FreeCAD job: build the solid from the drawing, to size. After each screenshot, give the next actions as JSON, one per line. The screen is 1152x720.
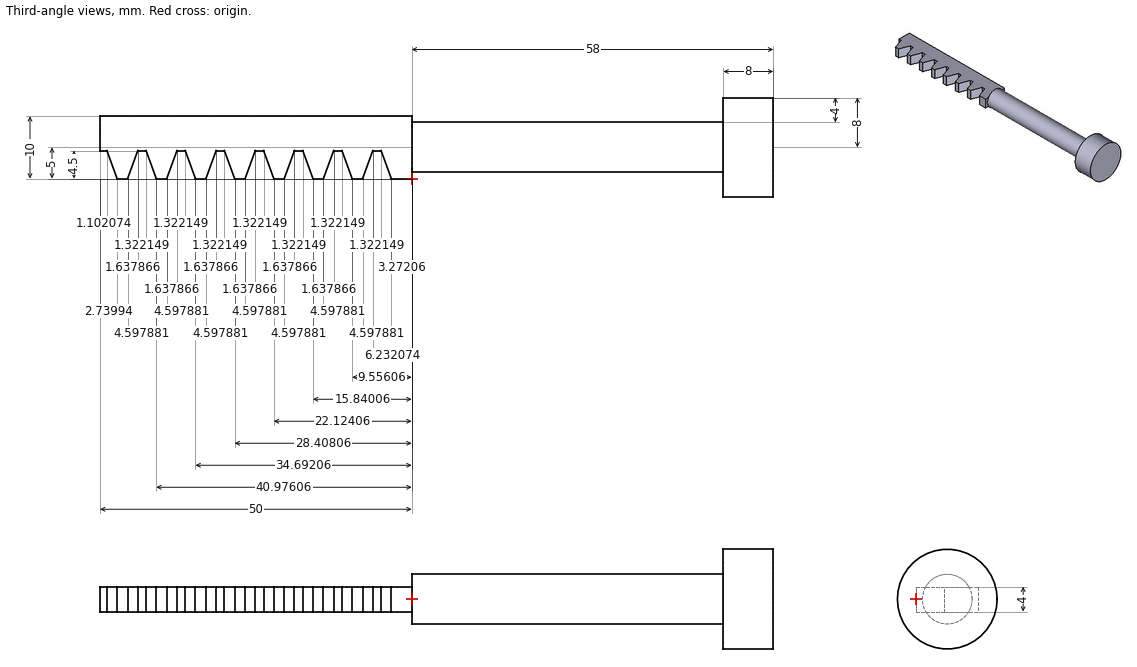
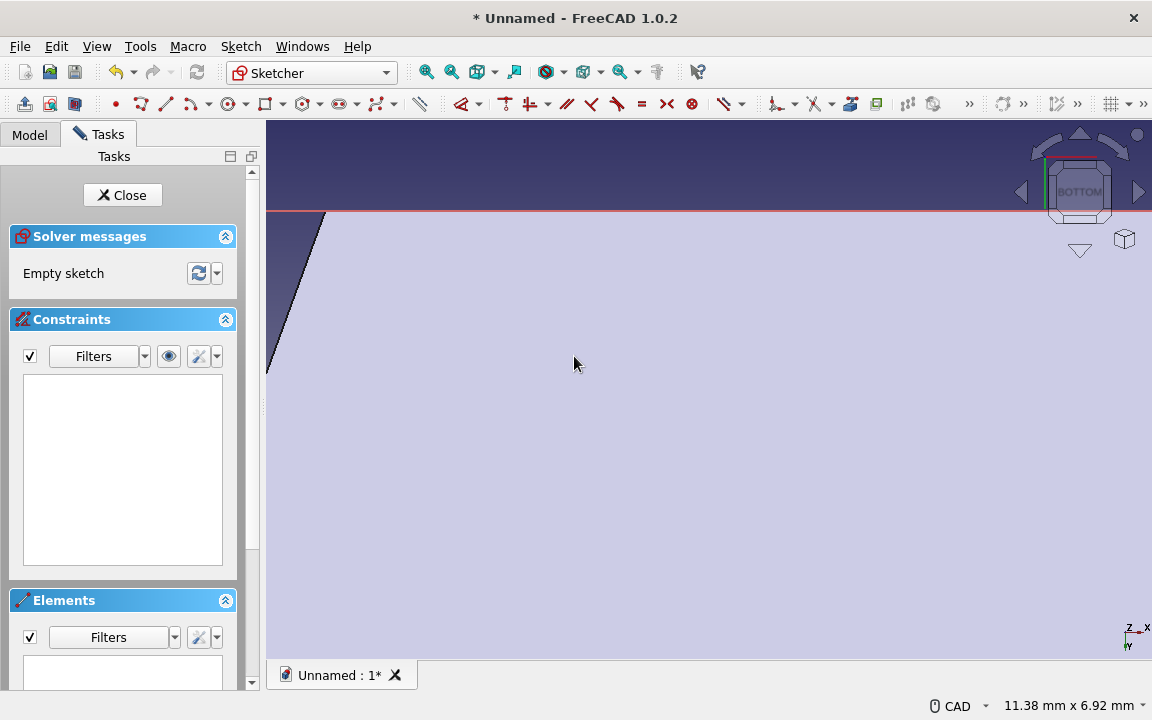
{"action": "left_click", "coordinate": [141, 104]}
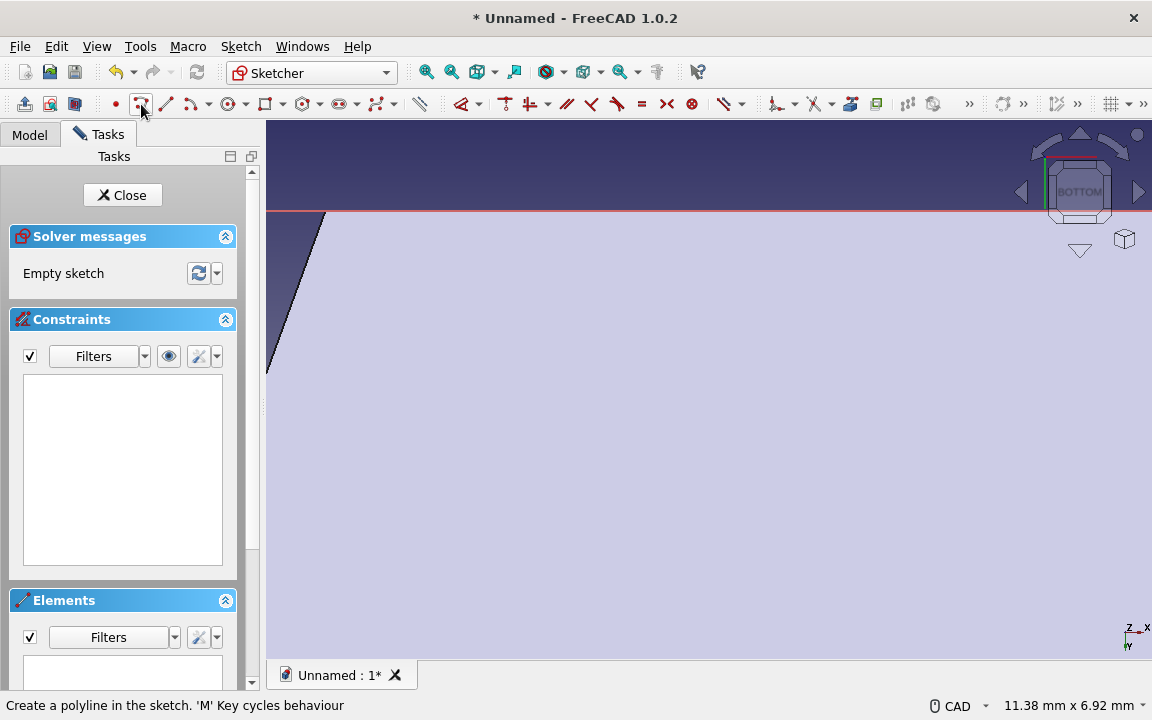
{"action": "left_click", "coordinate": [815, 211]}
{"action": "left_click", "coordinate": [457, 220]}
{"action": "left_click", "coordinate": [584, 562]}
{"action": "left_click", "coordinate": [687, 562]}
{"action": "left_click", "coordinate": [815, 211]}
{"action": "key", "text": "Escape"}
{"action": "key", "text": "Escape"}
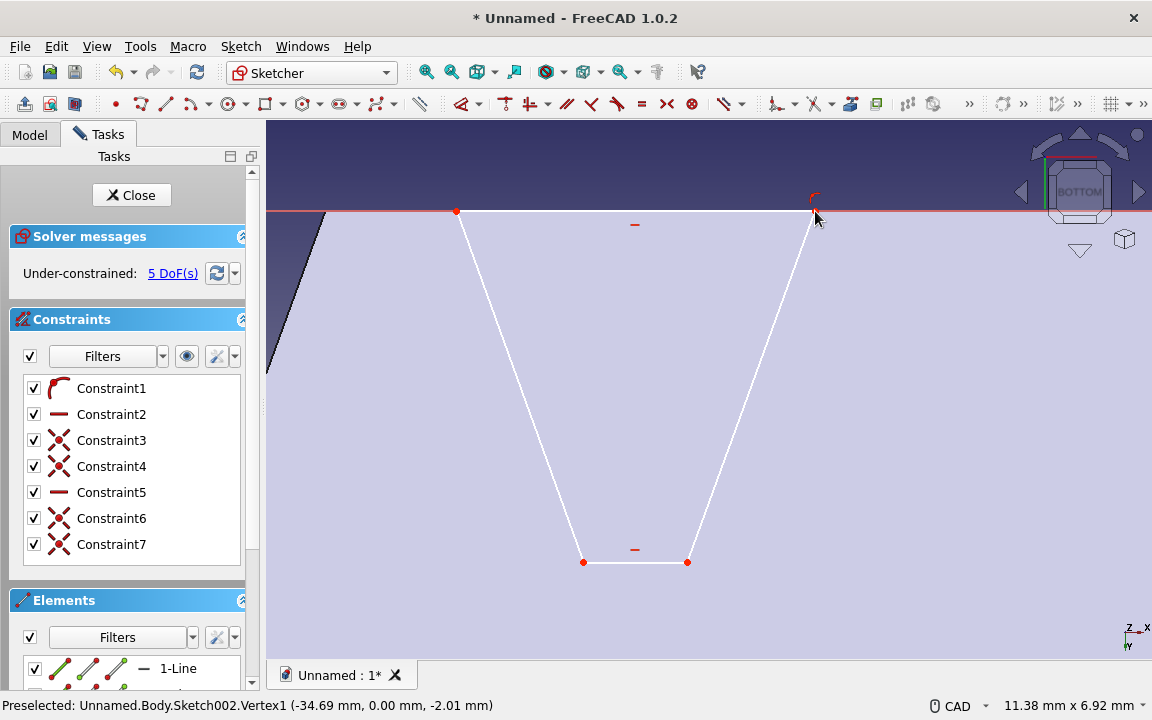
{"action": "left_click", "coordinate": [460, 104]}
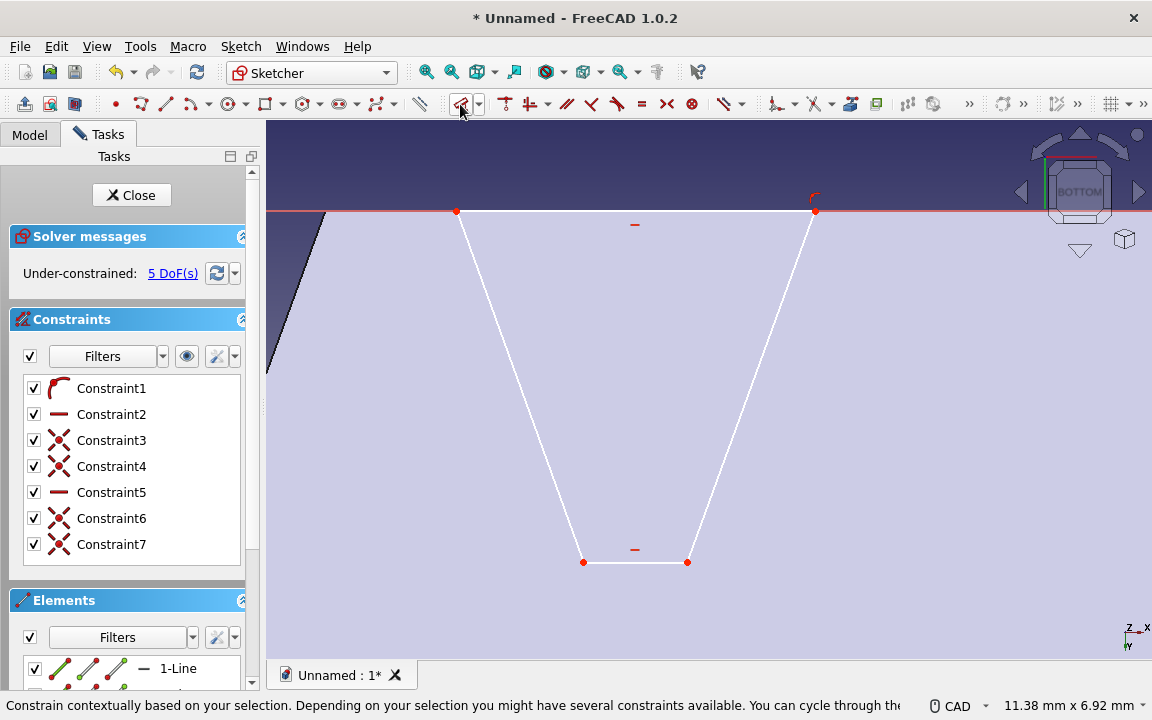
{"action": "left_click", "coordinate": [584, 563]}
{"action": "left_click", "coordinate": [550, 387]}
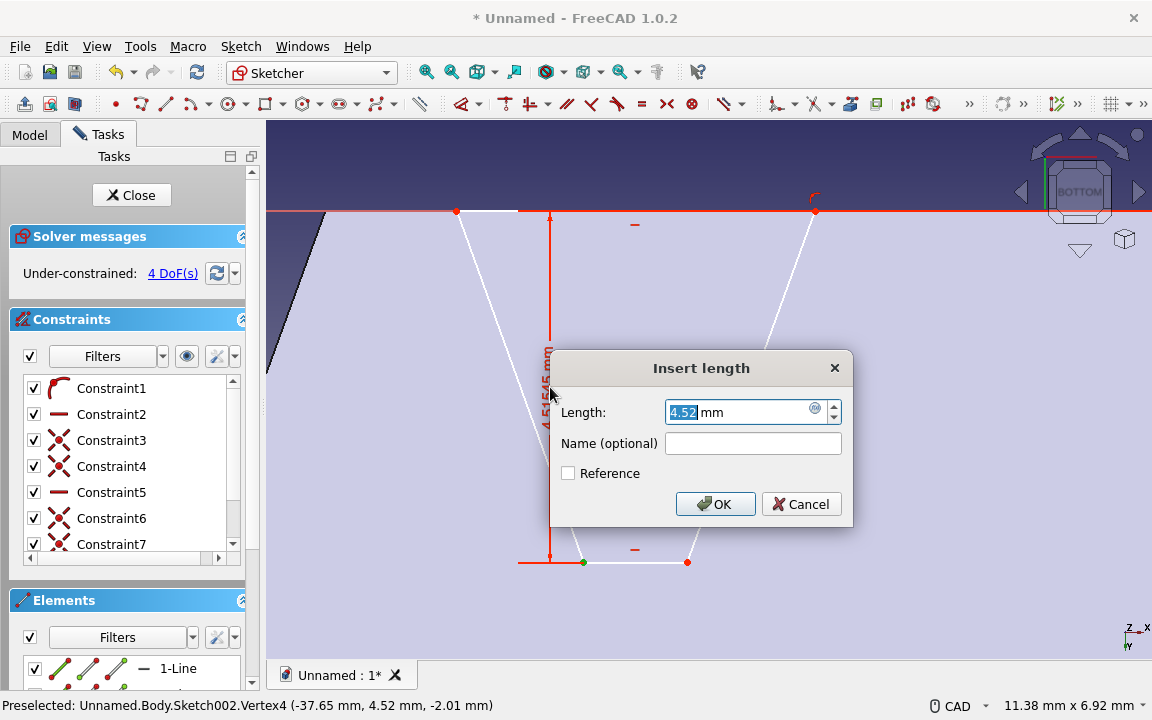
{"action": "type", "text": "4.5"}
{"action": "key", "text": "Return"}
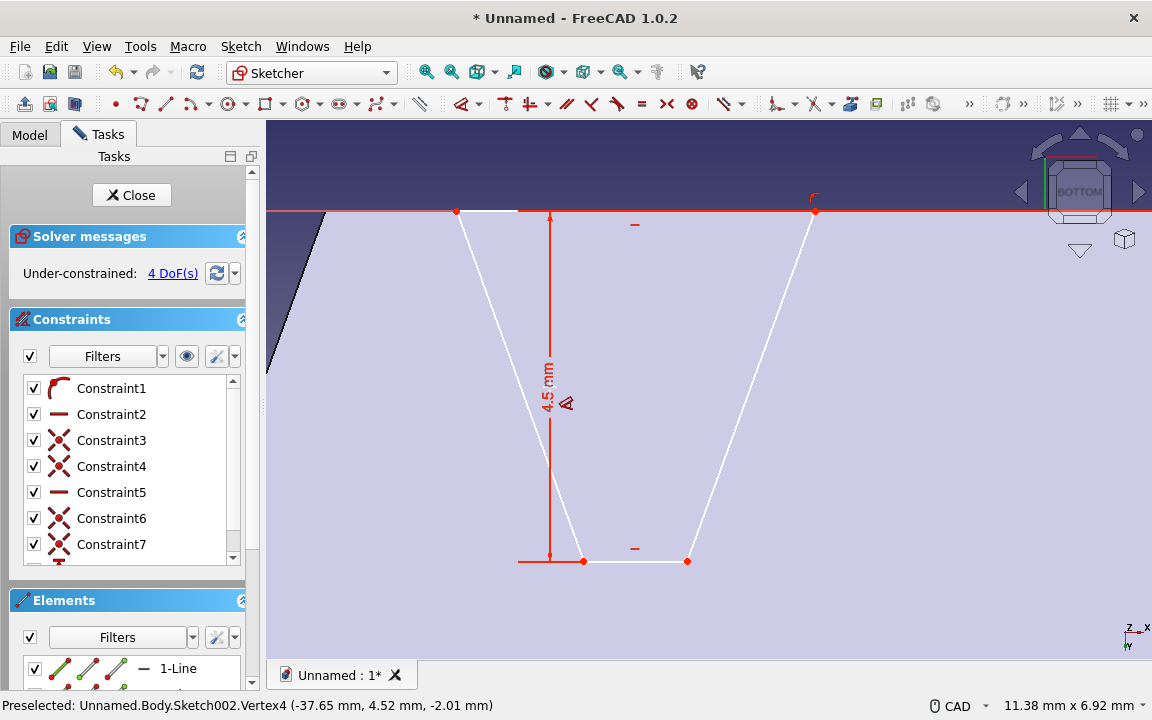
{"action": "left_click", "coordinate": [708, 211]}
{"action": "left_click", "coordinate": [636, 177]}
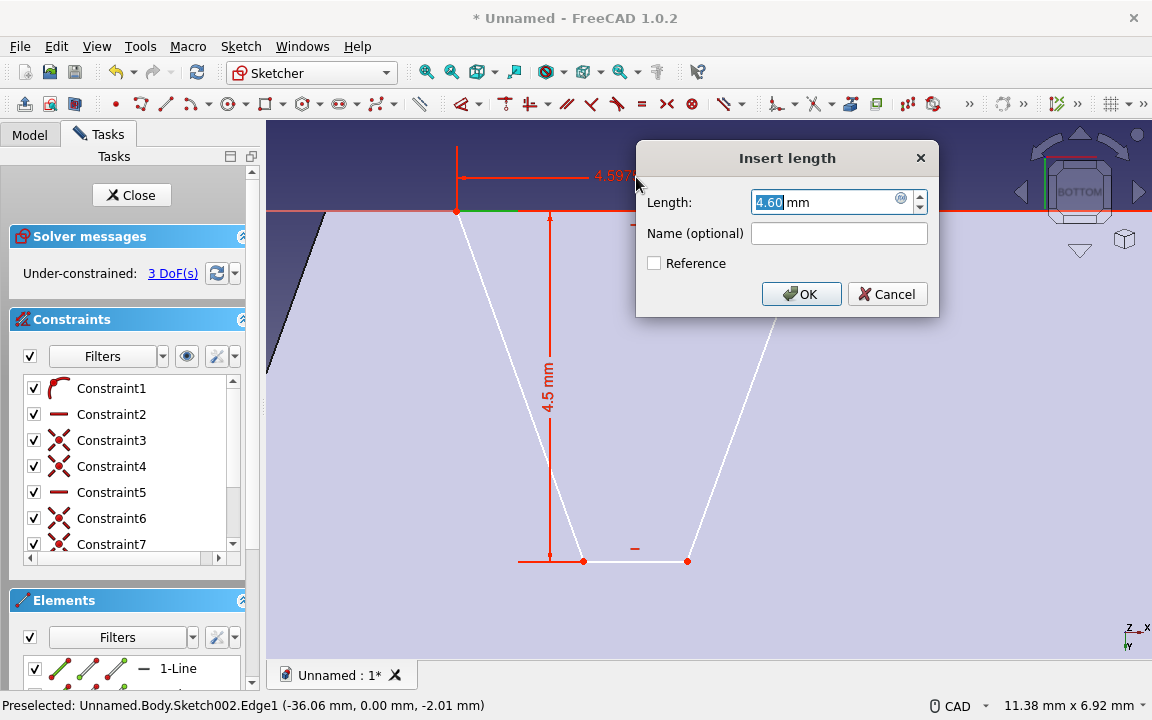
{"action": "type", "text": "4.597881"}
{"action": "key", "text": "Return"}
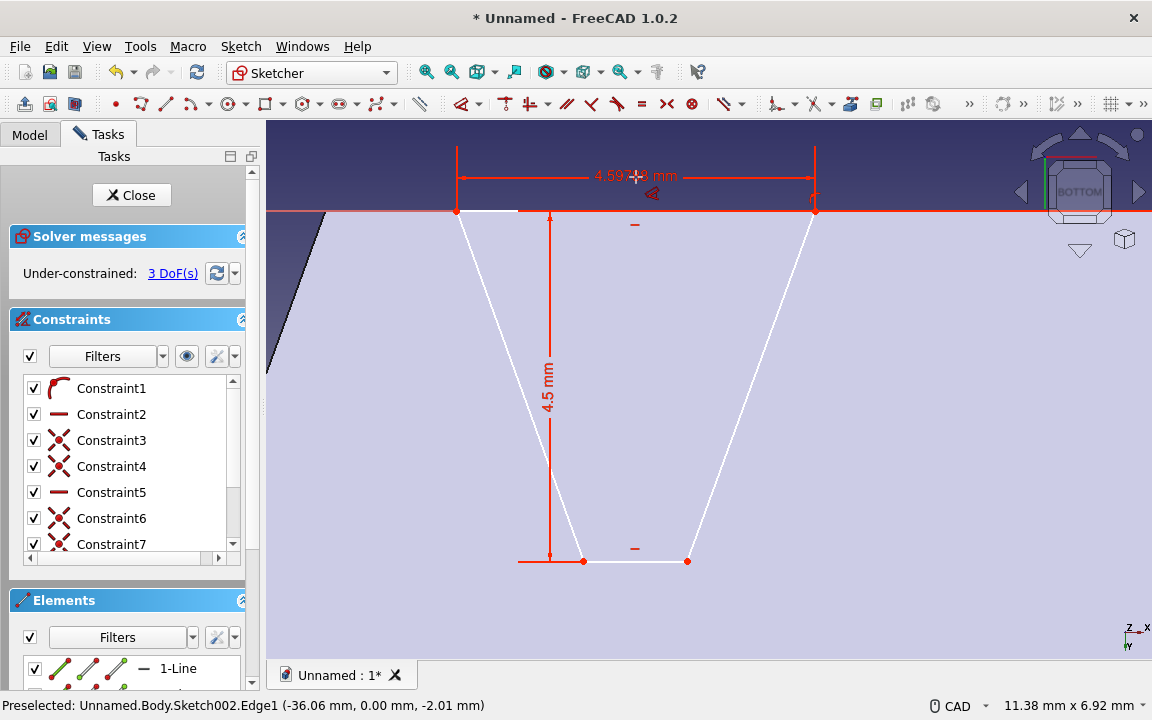
{"action": "left_click", "coordinate": [615, 562]}
{"action": "left_click", "coordinate": [636, 596]}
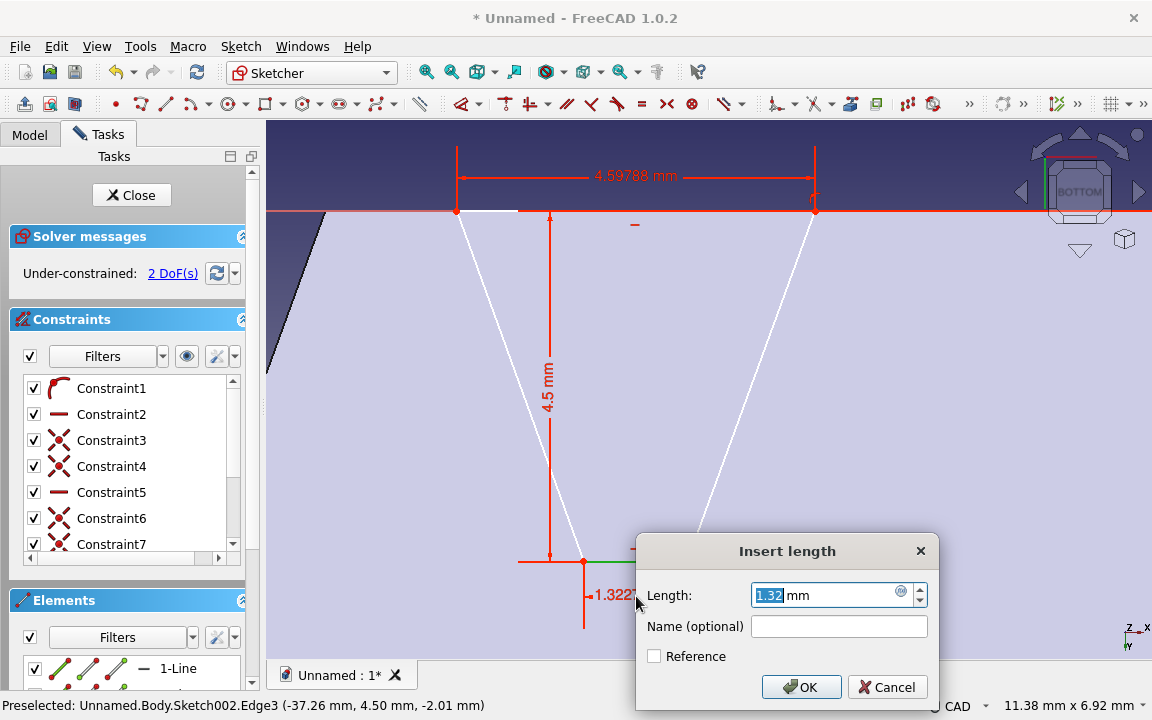
{"action": "type", "text": "1.322149"}
{"action": "key", "text": "Return"}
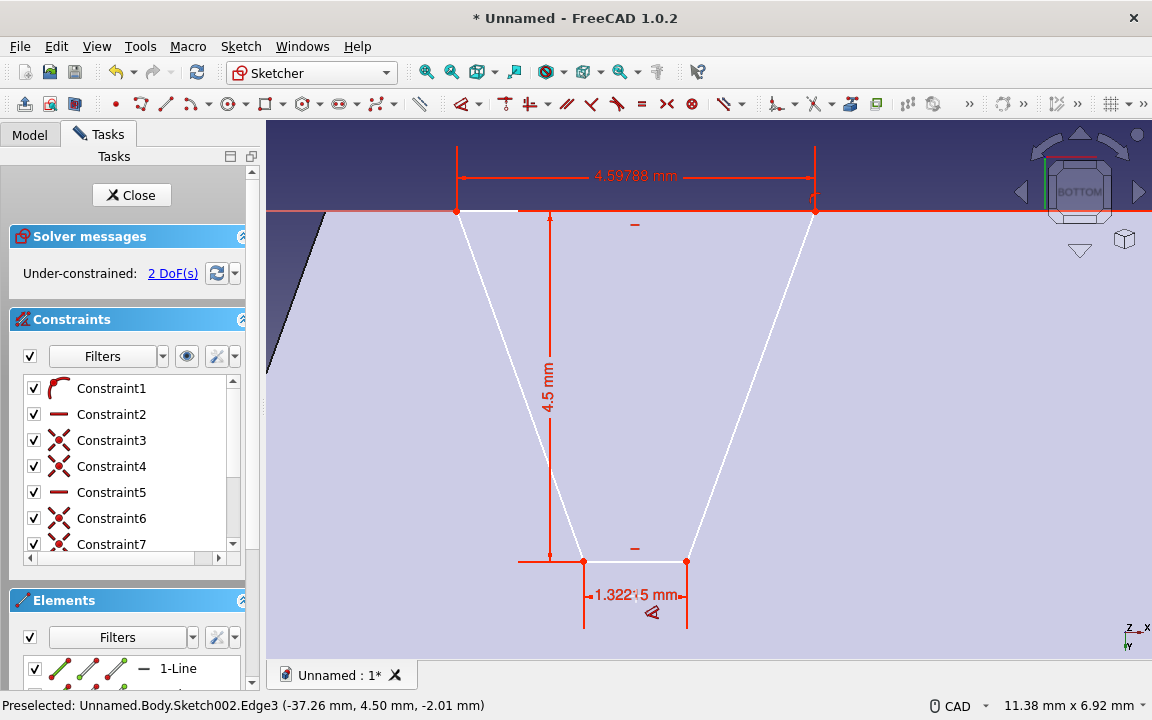
{"action": "left_click", "coordinate": [815, 211]}
{"action": "left_click", "coordinate": [901, 177]}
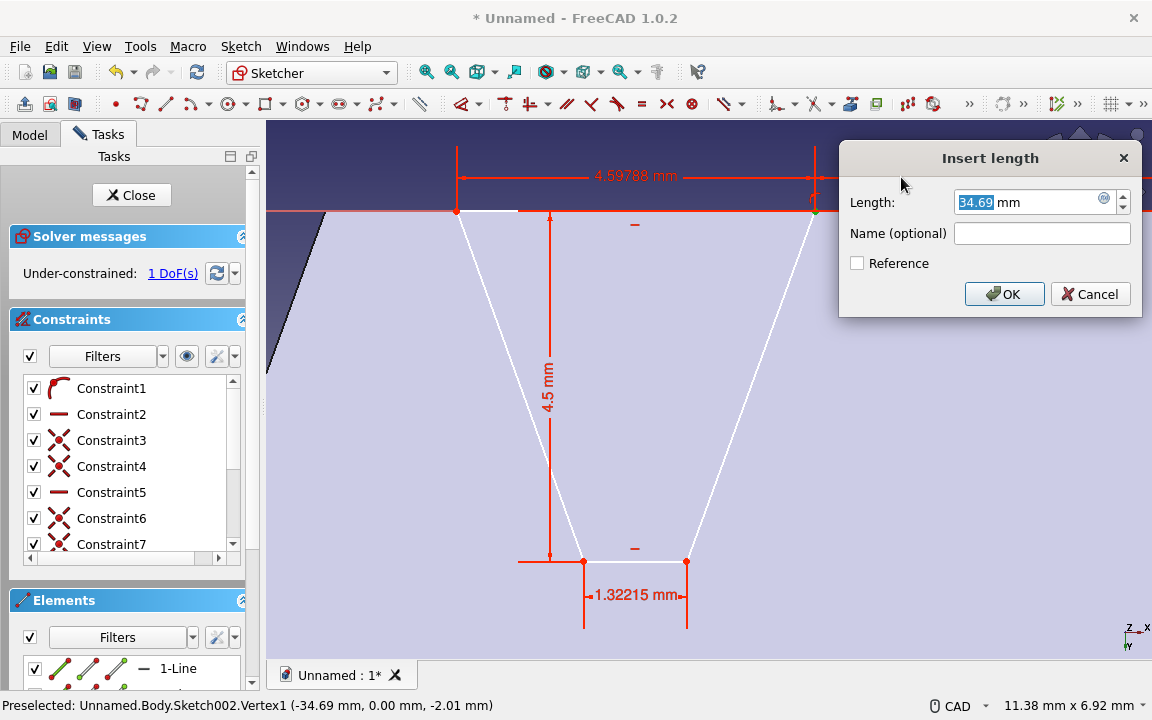
{"action": "type", "text": "34.69206"}
{"action": "key", "text": "Return"}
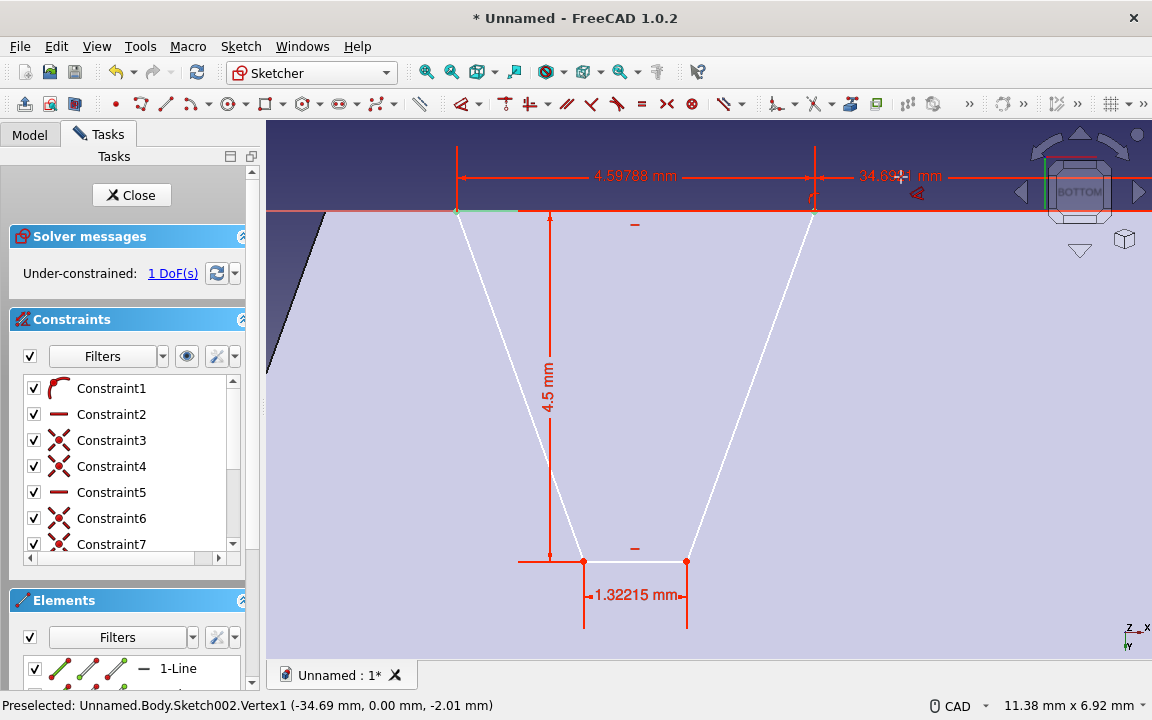
{"action": "left_click", "coordinate": [495, 317]}
{"action": "left_click", "coordinate": [520, 596]}